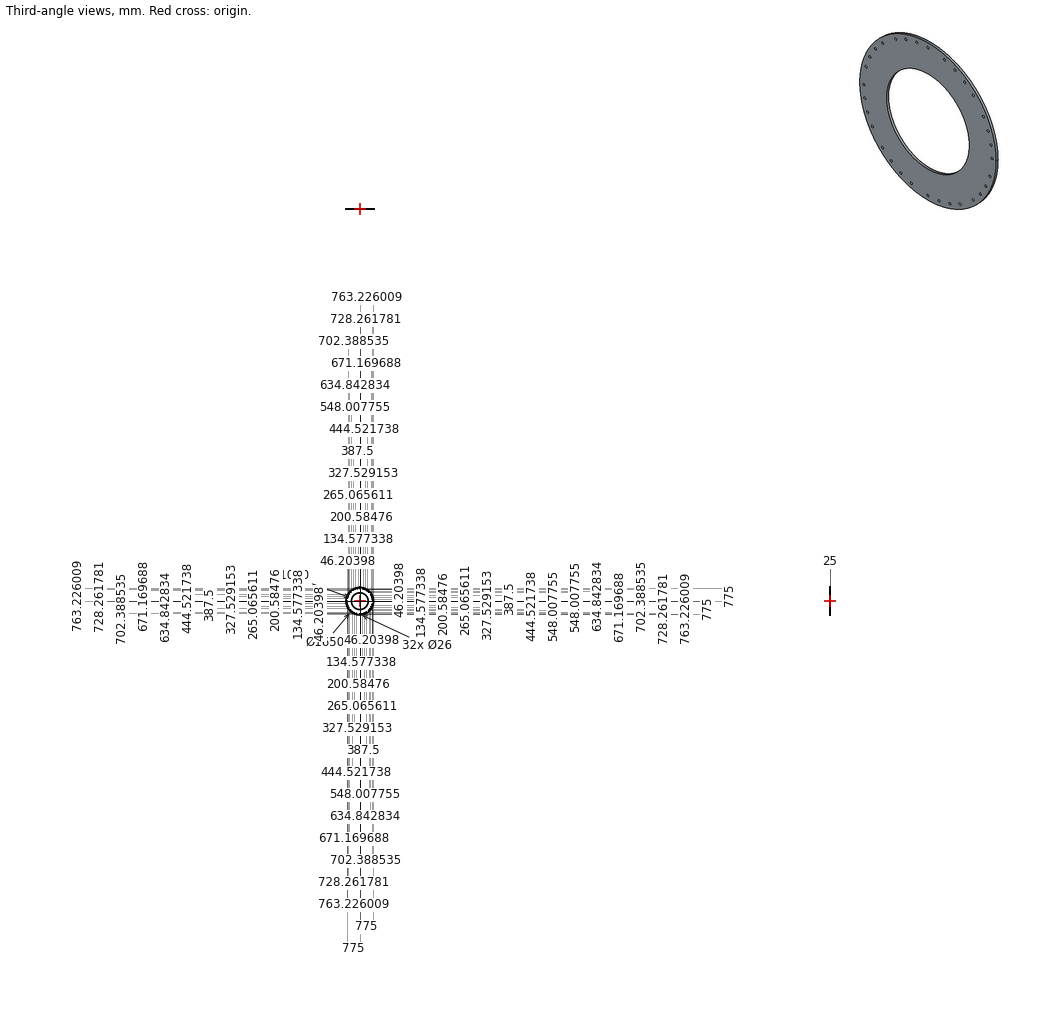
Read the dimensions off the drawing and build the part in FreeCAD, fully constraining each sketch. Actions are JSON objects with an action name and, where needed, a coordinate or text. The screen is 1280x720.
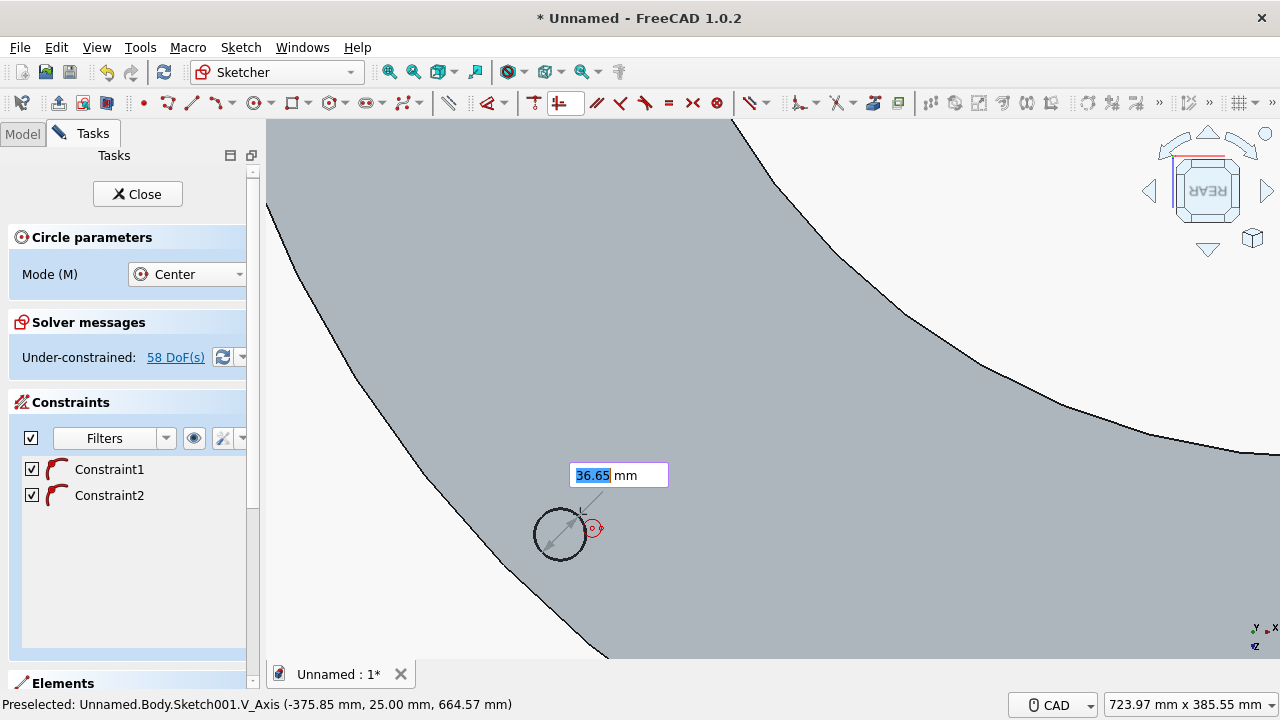
{"action": "left_click", "coordinate": [576, 513]}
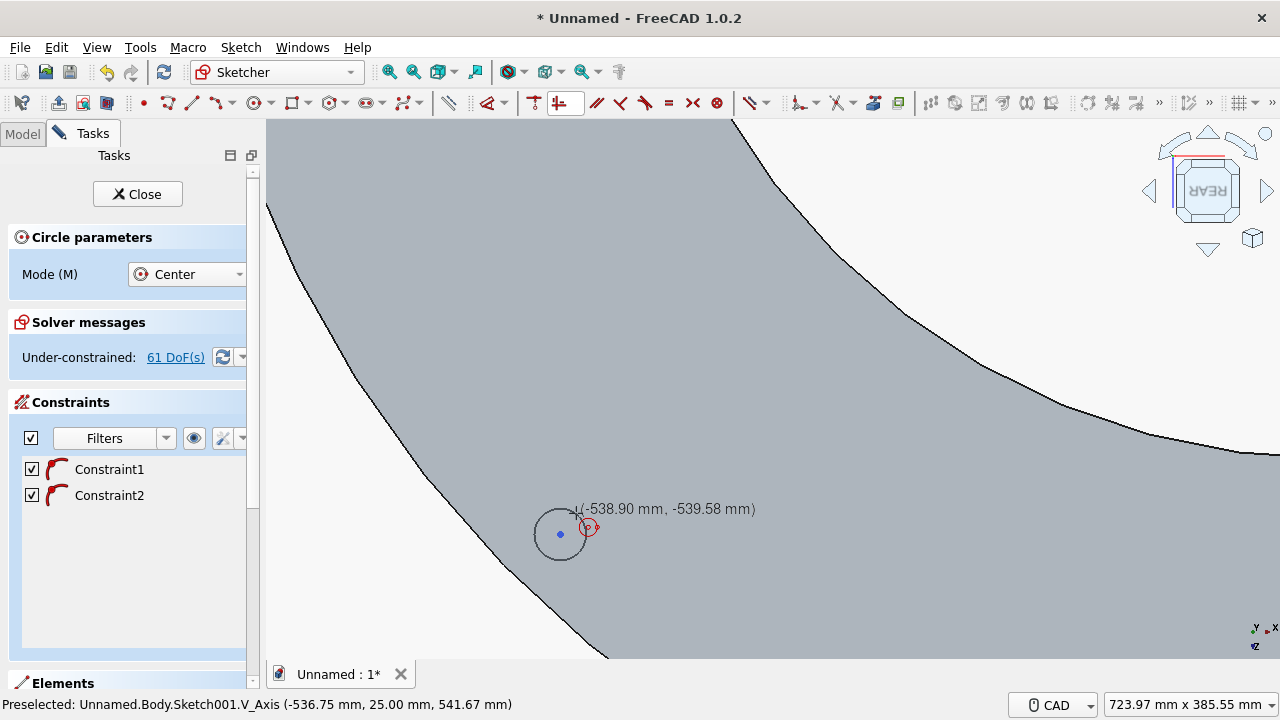
{"action": "scroll", "coordinate": [442, 381], "scroll_direction": "up", "scroll_amount": 2}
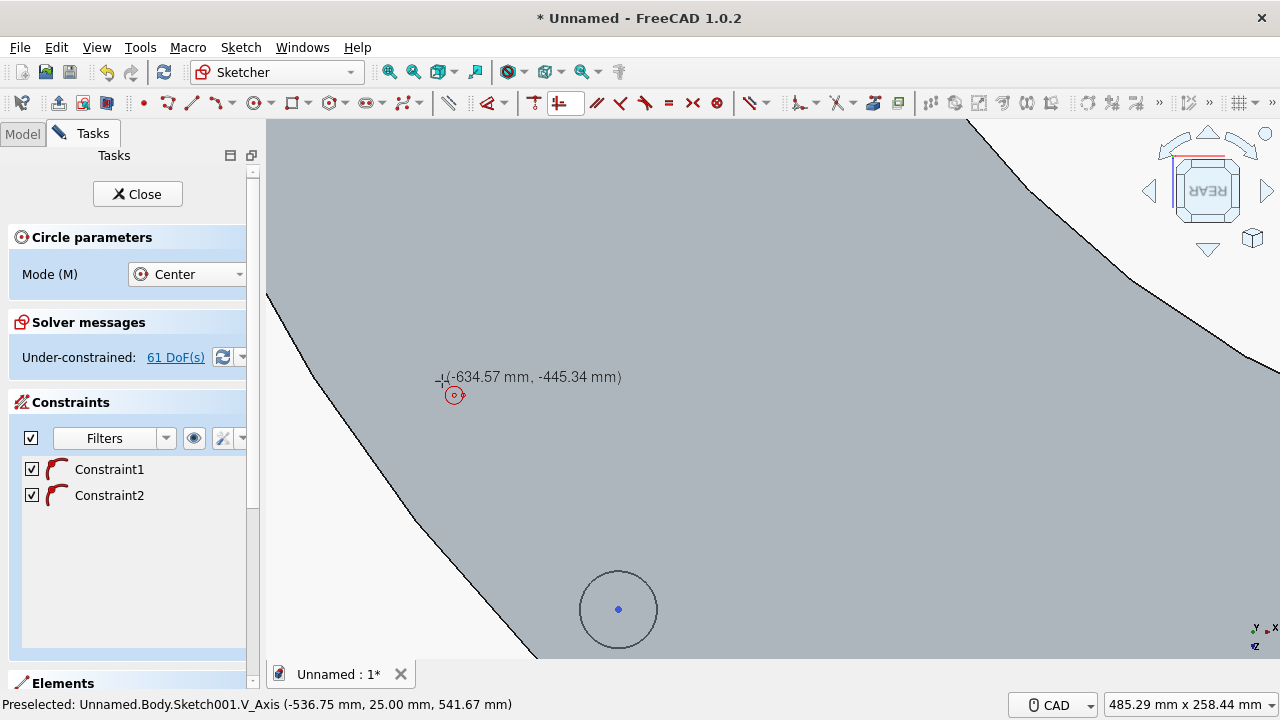
{"action": "scroll", "coordinate": [572, 506], "scroll_direction": "down", "scroll_amount": 11}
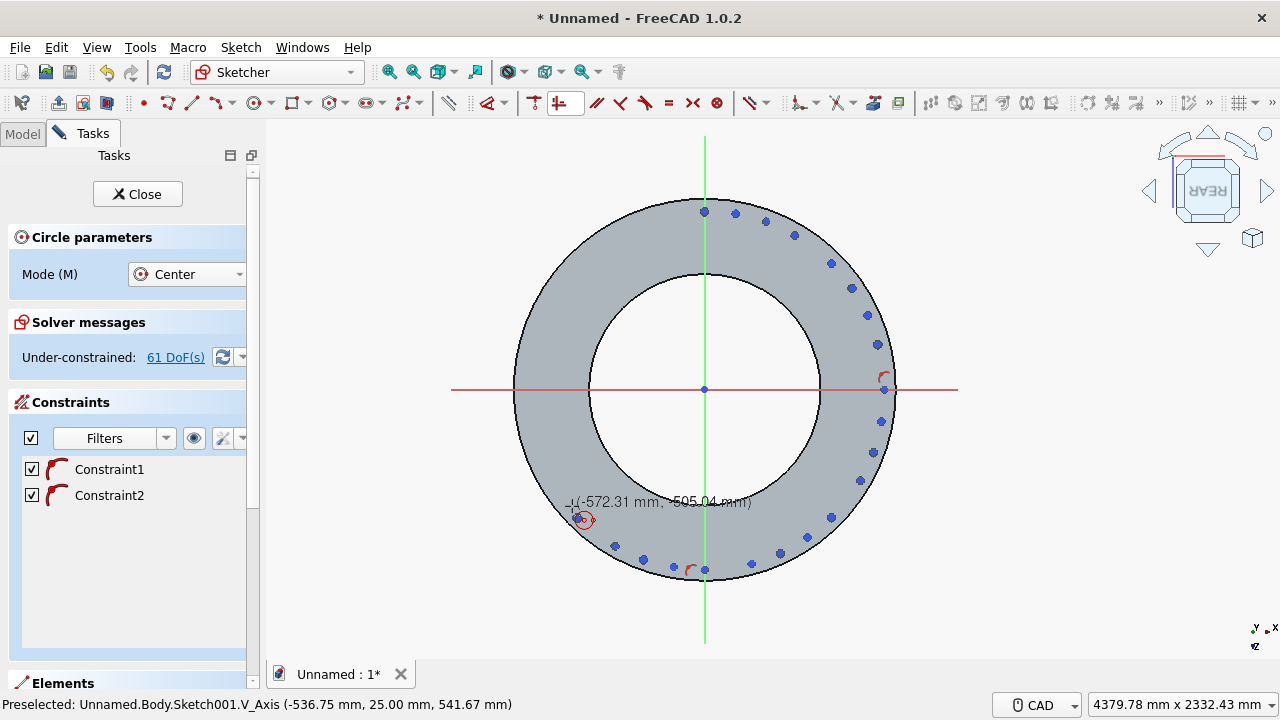
{"action": "left_click", "coordinate": [558, 493]}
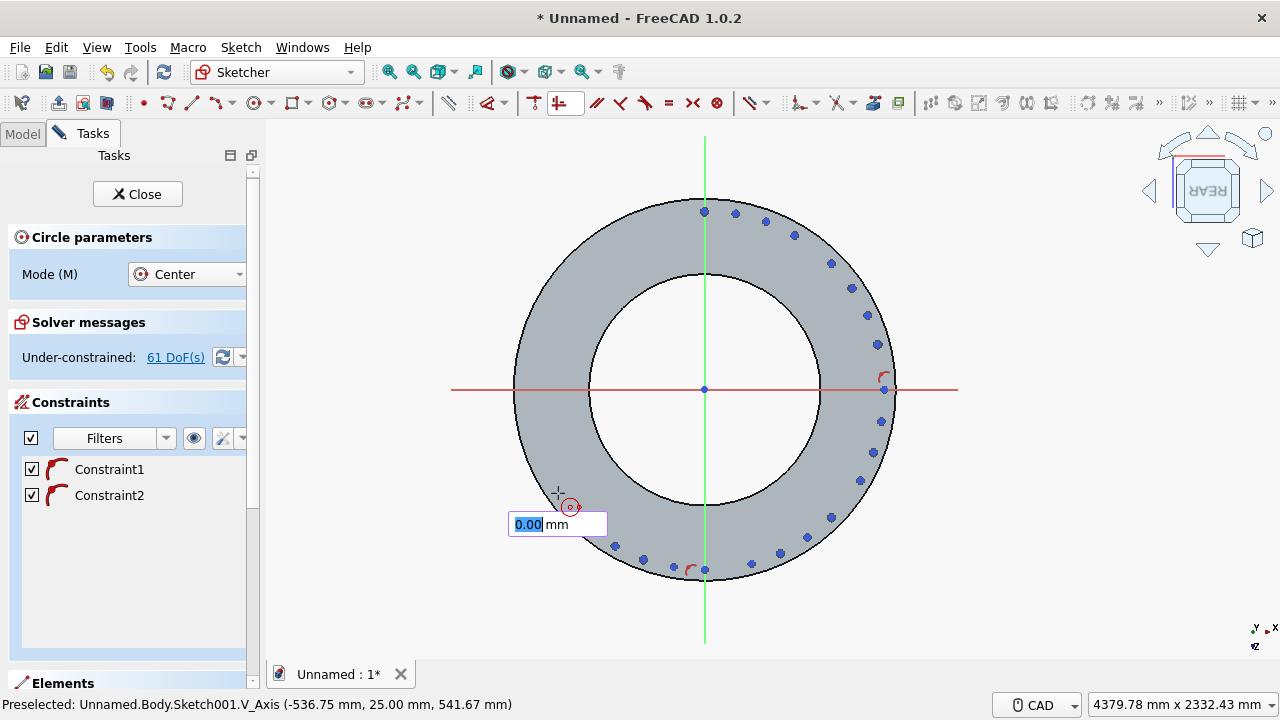
{"action": "scroll", "coordinate": [560, 491], "scroll_direction": "up", "scroll_amount": 9}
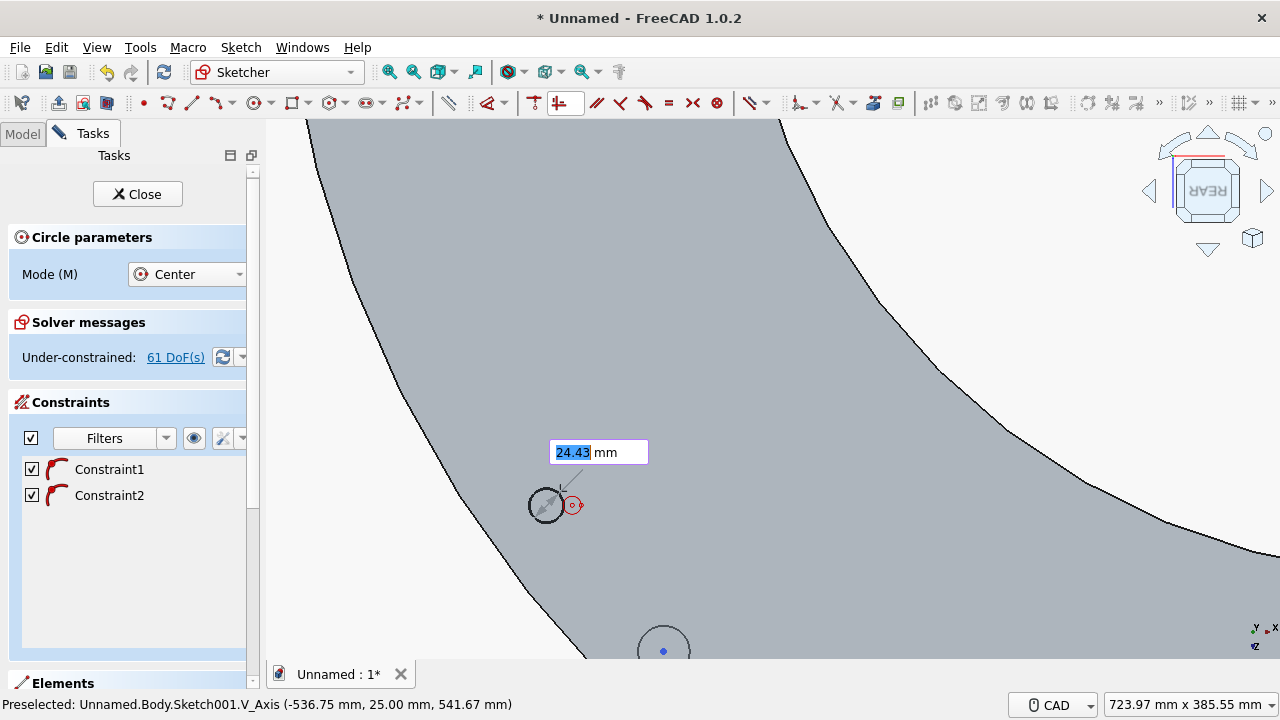
{"action": "left_click", "coordinate": [558, 485]}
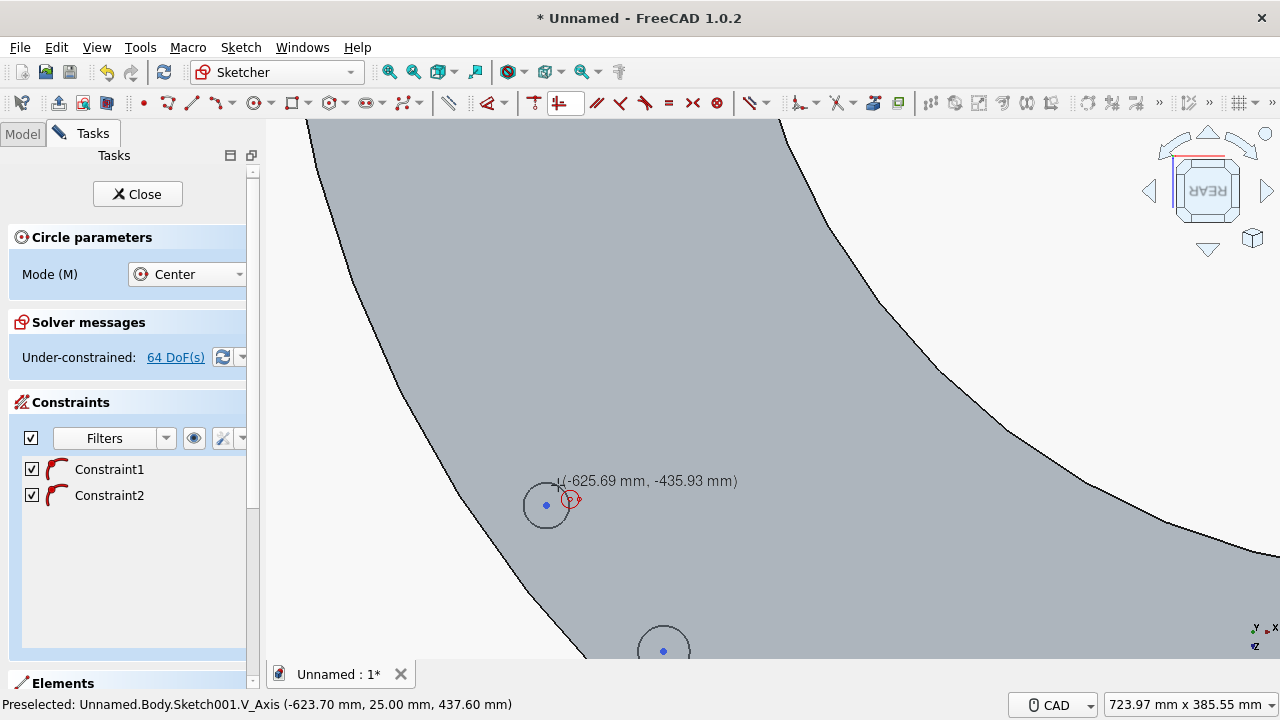
{"action": "scroll", "coordinate": [451, 334], "scroll_direction": "up", "scroll_amount": 2}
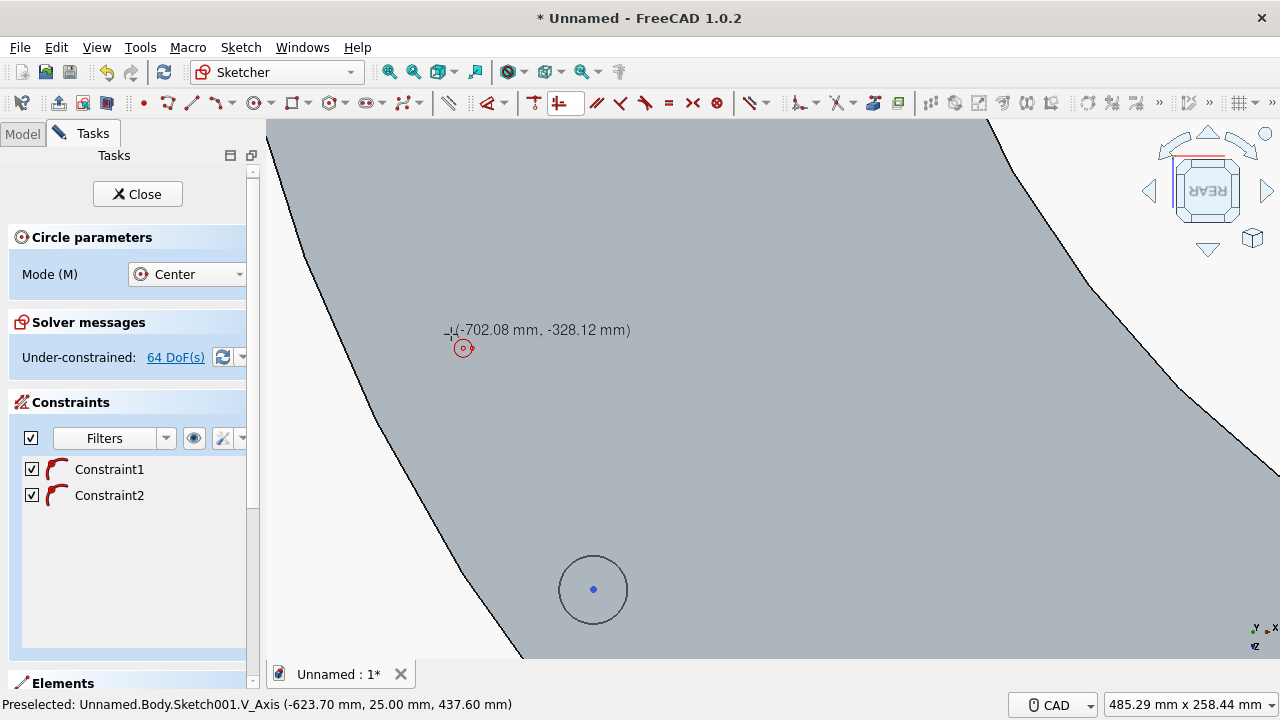
{"action": "scroll", "coordinate": [553, 481], "scroll_direction": "down", "scroll_amount": 11}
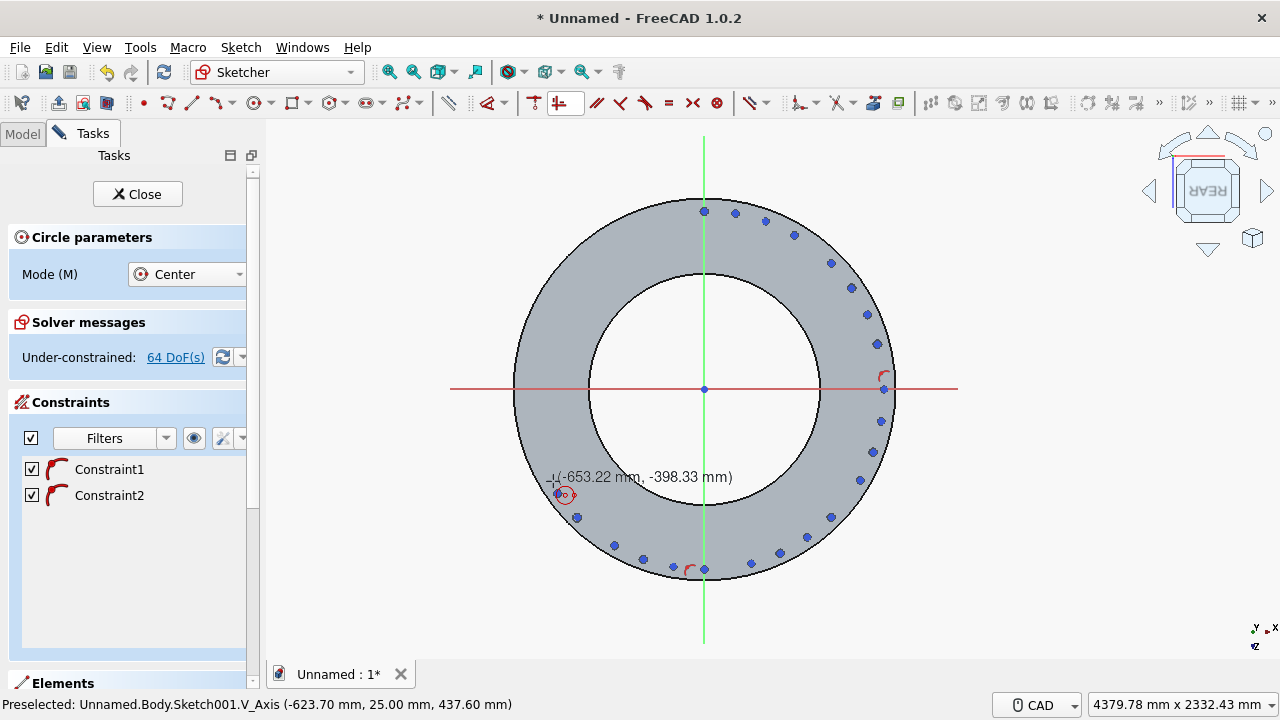
{"action": "left_click", "coordinate": [542, 465]}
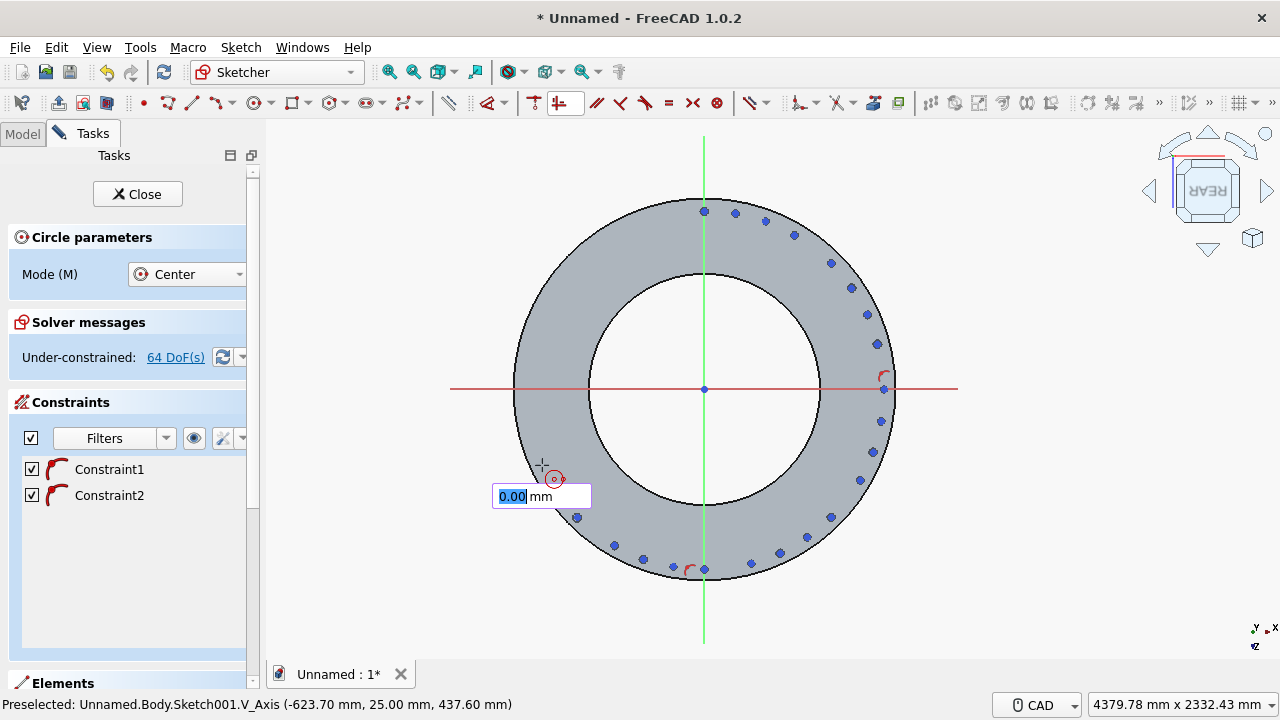
{"action": "scroll", "coordinate": [544, 463], "scroll_direction": "up", "scroll_amount": 9}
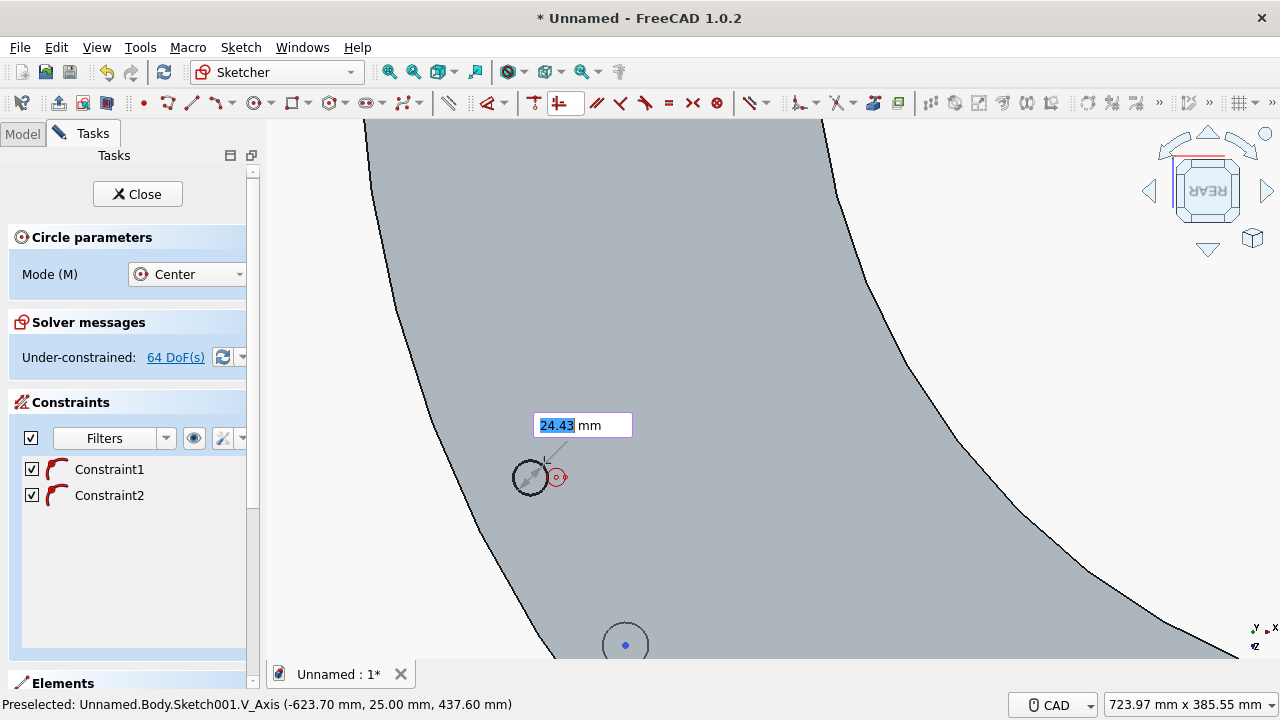
{"action": "left_click", "coordinate": [543, 461]}